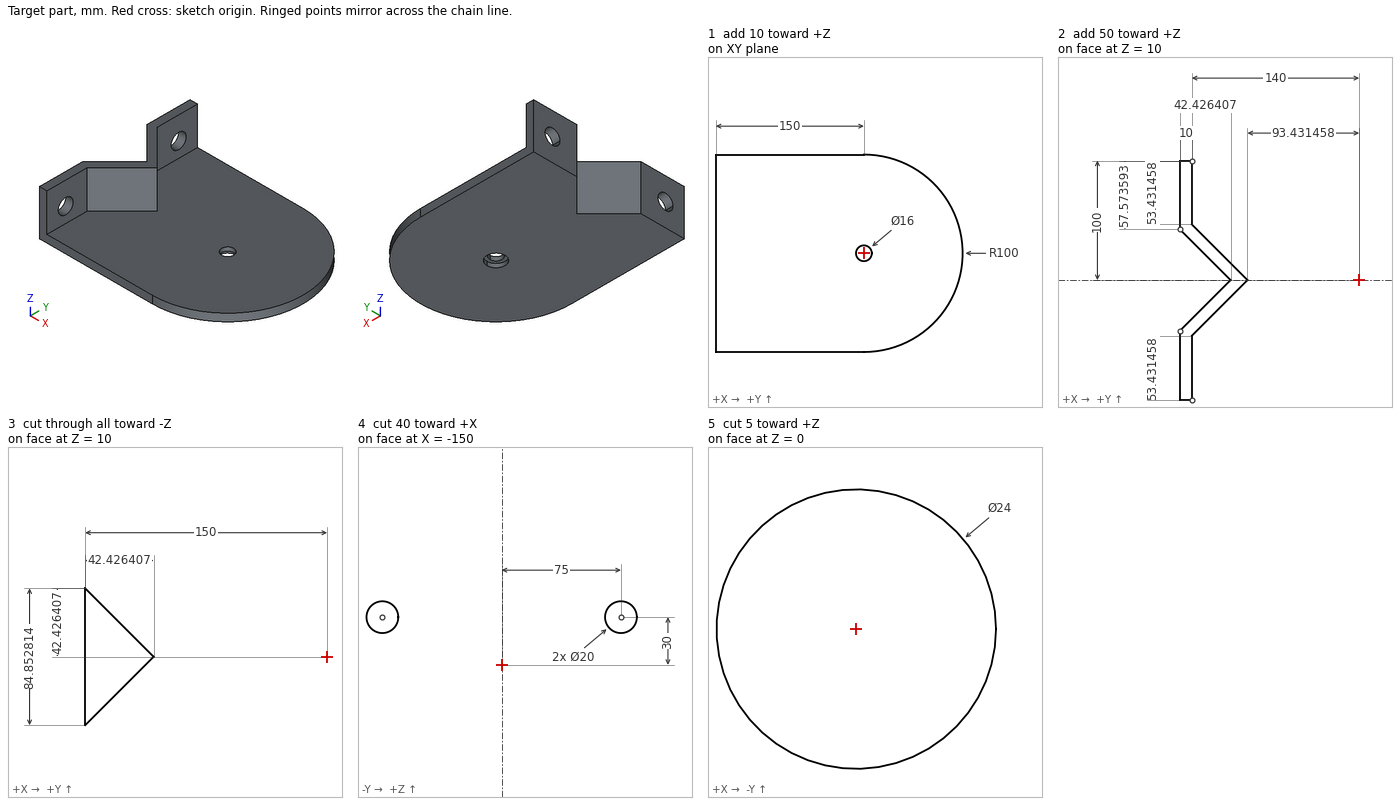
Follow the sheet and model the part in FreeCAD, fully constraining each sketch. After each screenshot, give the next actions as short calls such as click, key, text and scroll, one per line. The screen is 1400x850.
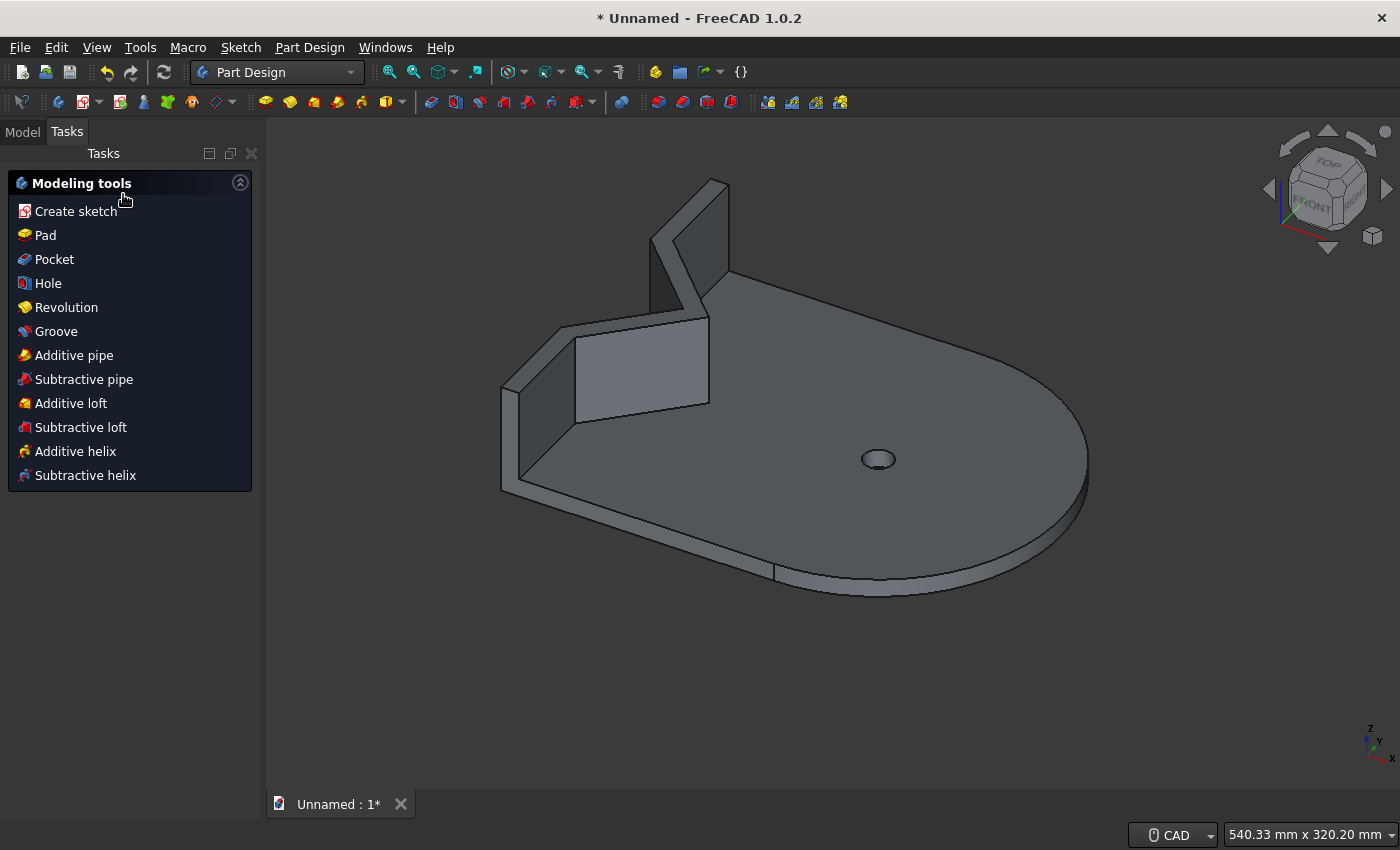
click(432, 102)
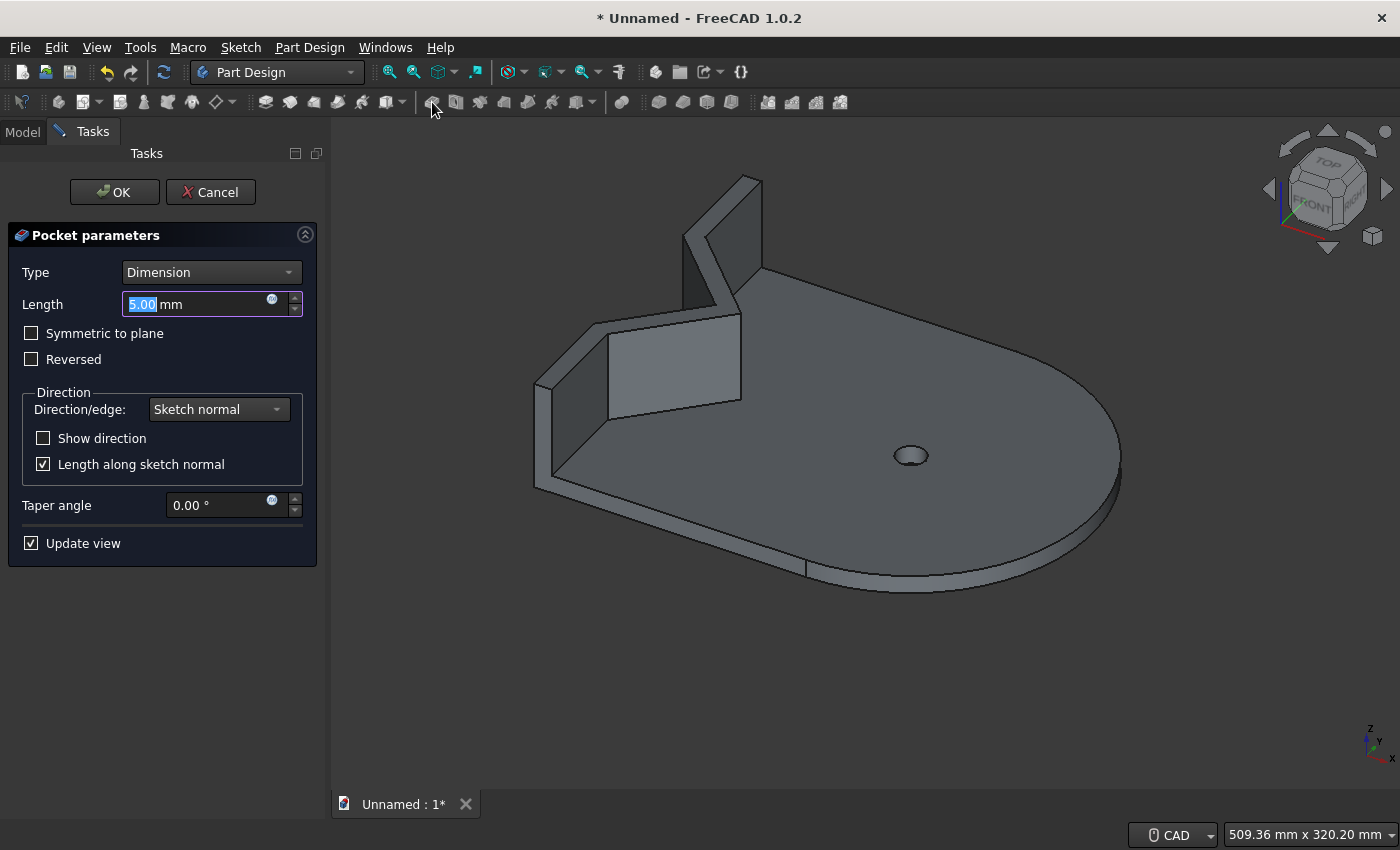
click(212, 272)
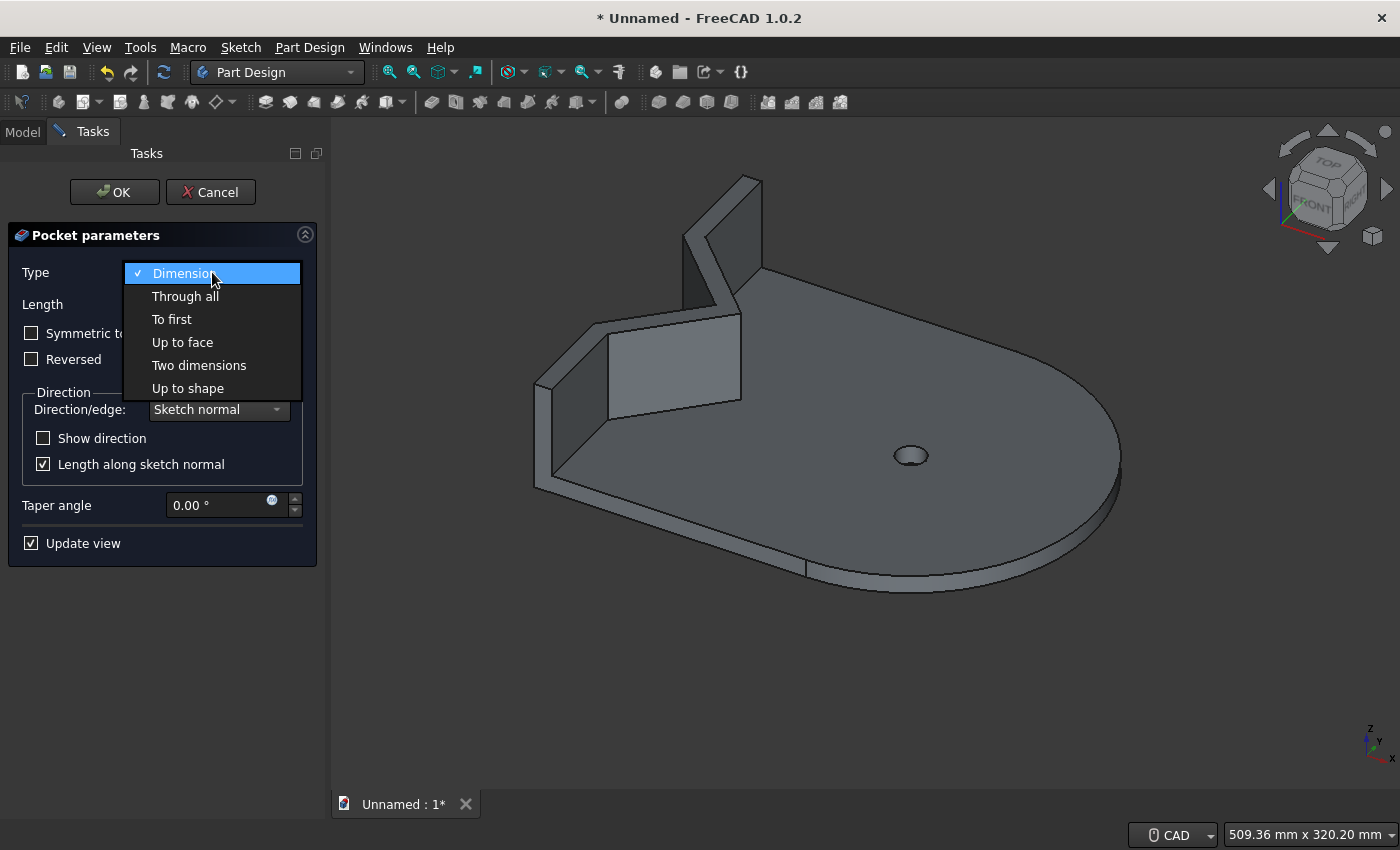
click(212, 296)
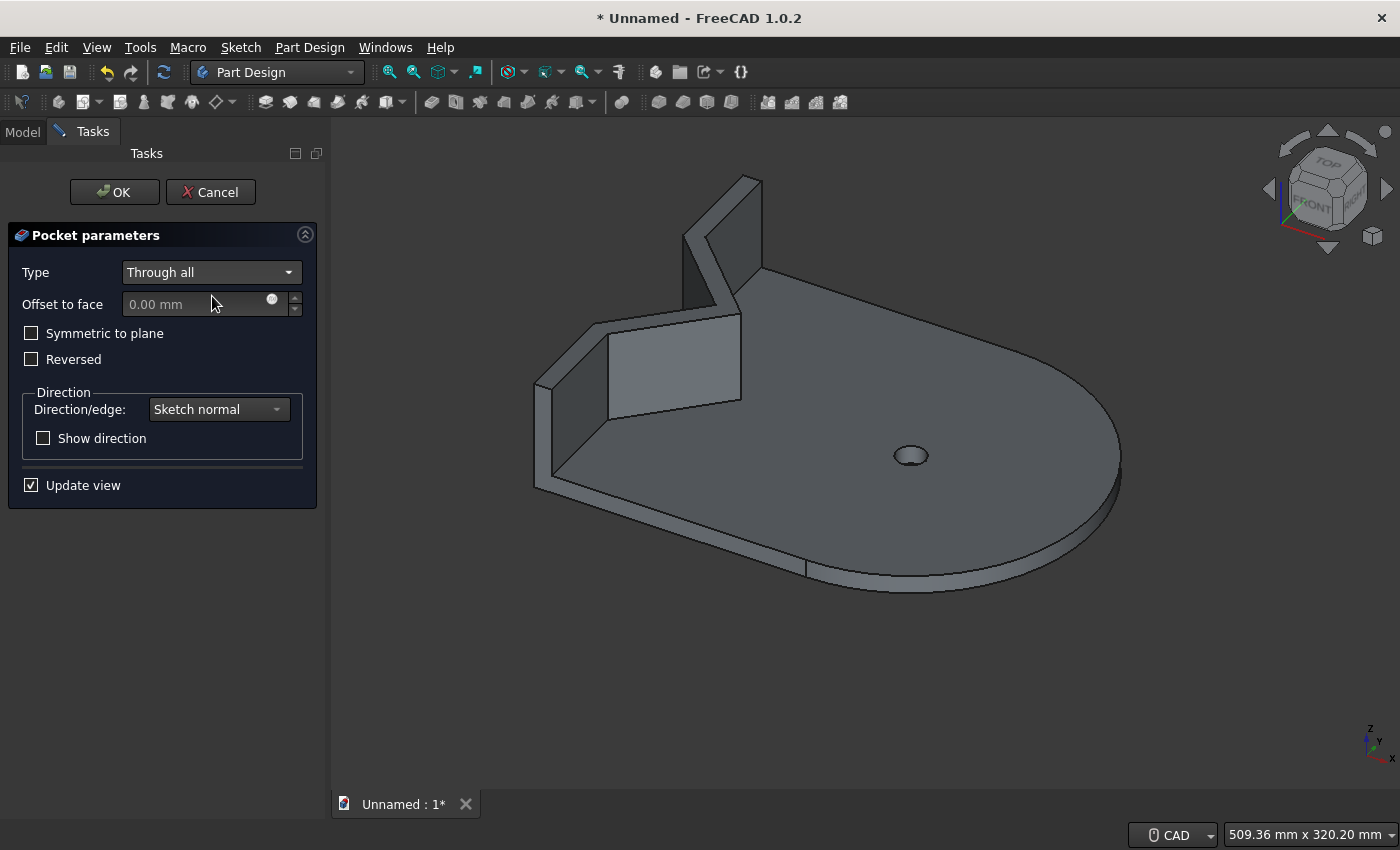
click(115, 192)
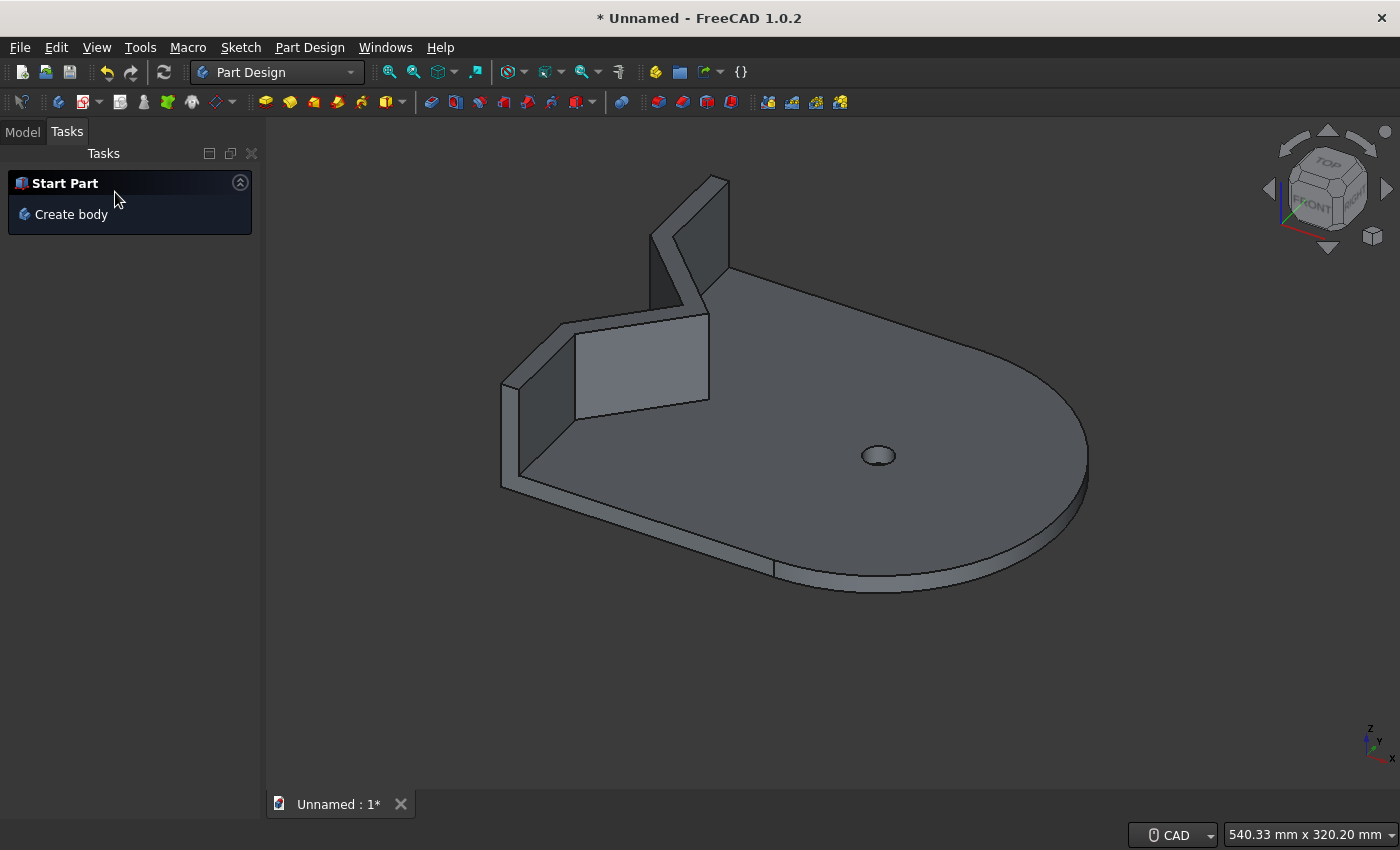
key(6)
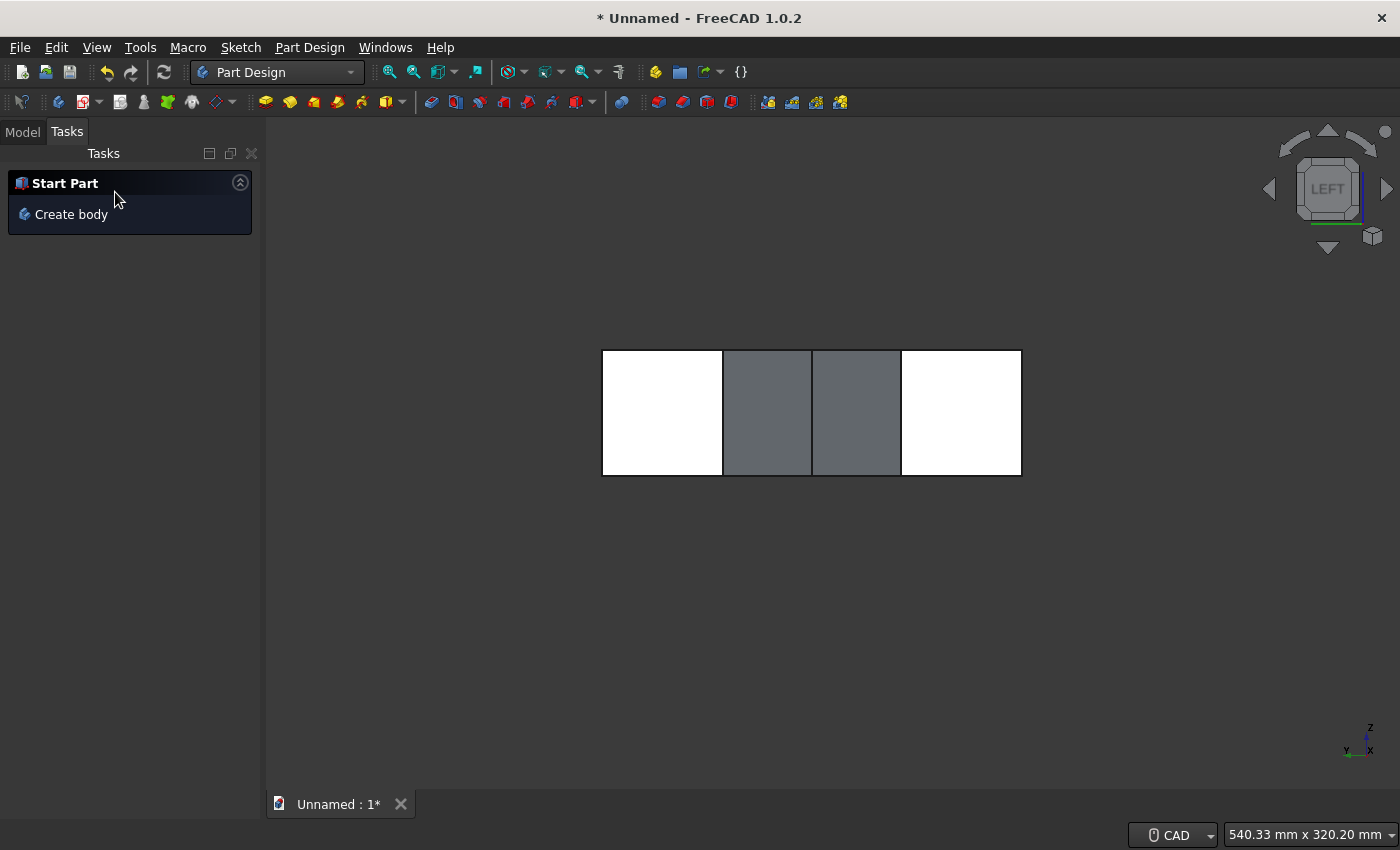
key(v)
key(f)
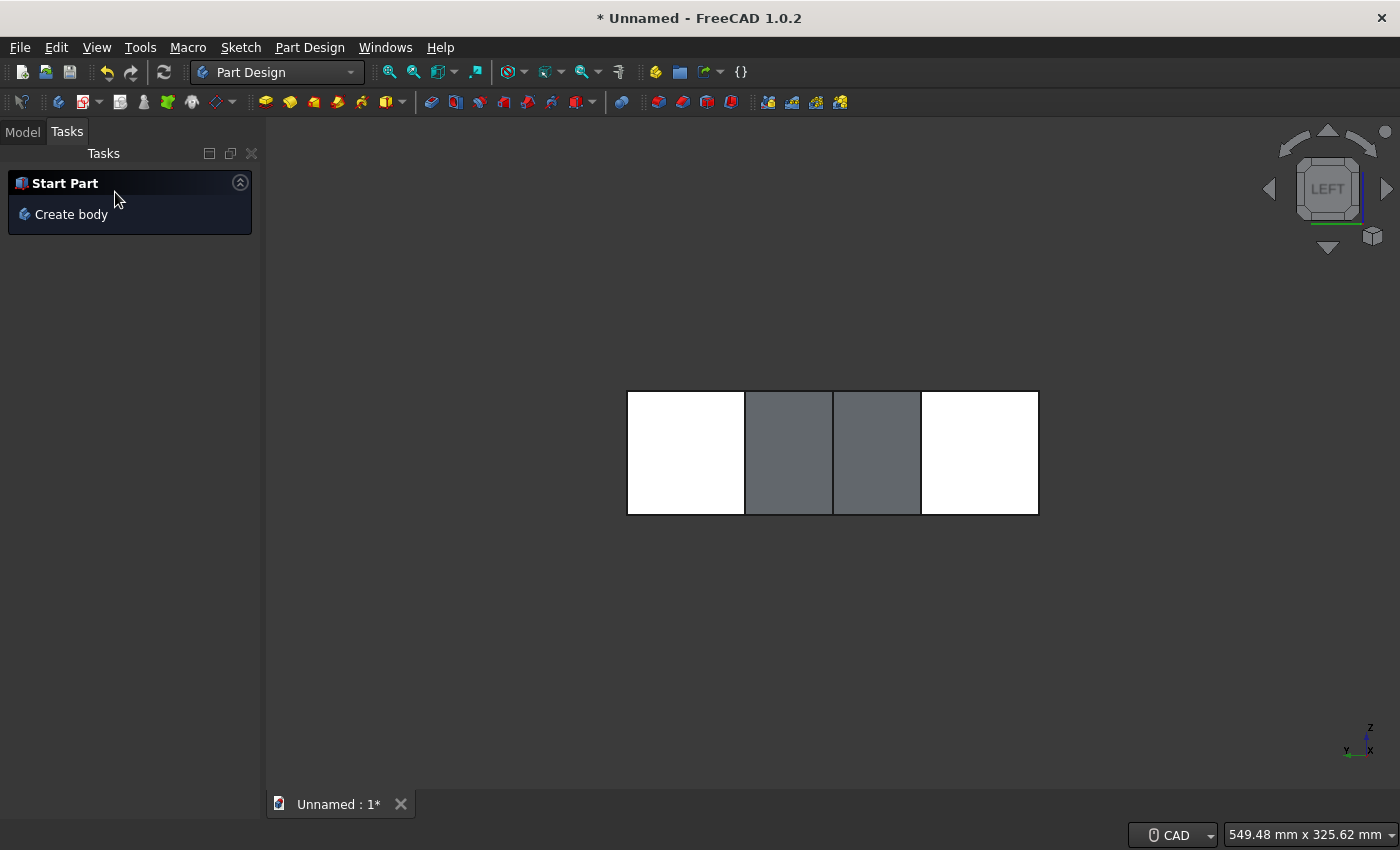
click(980, 452)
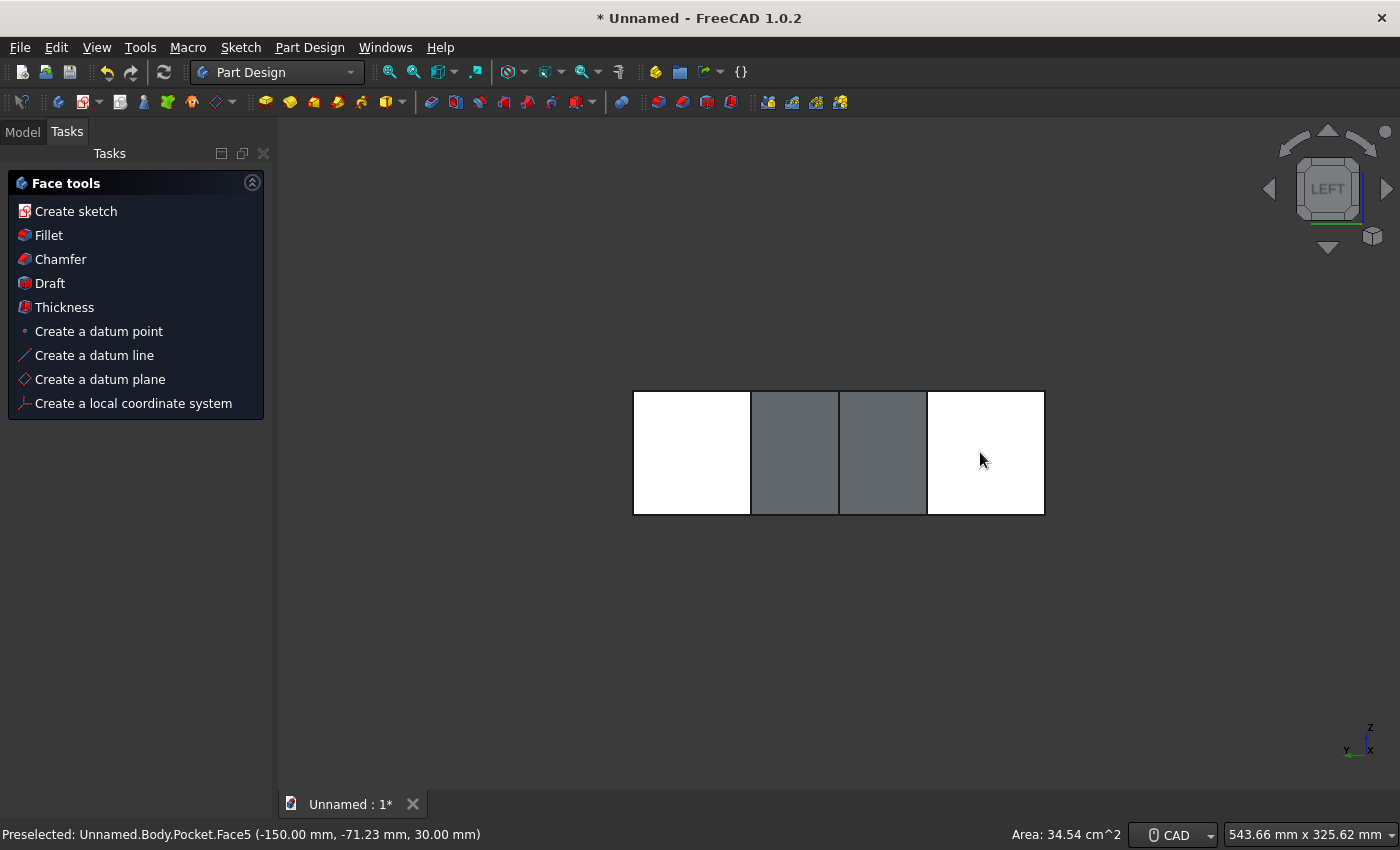
click(84, 102)